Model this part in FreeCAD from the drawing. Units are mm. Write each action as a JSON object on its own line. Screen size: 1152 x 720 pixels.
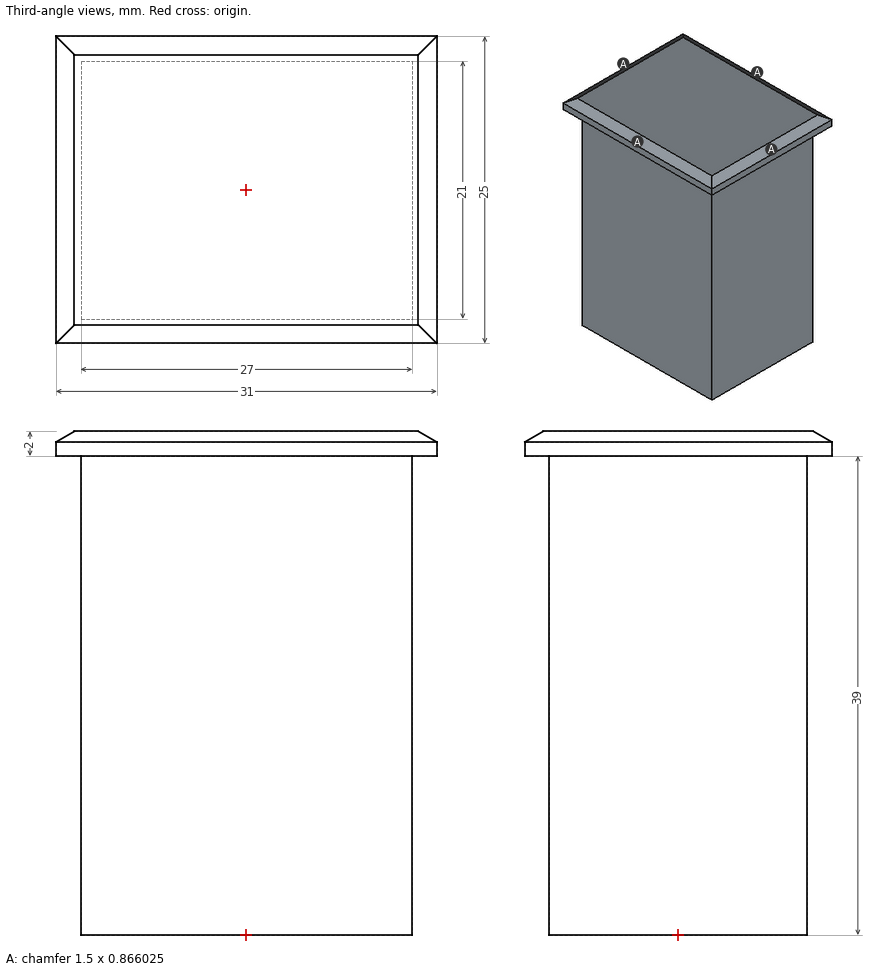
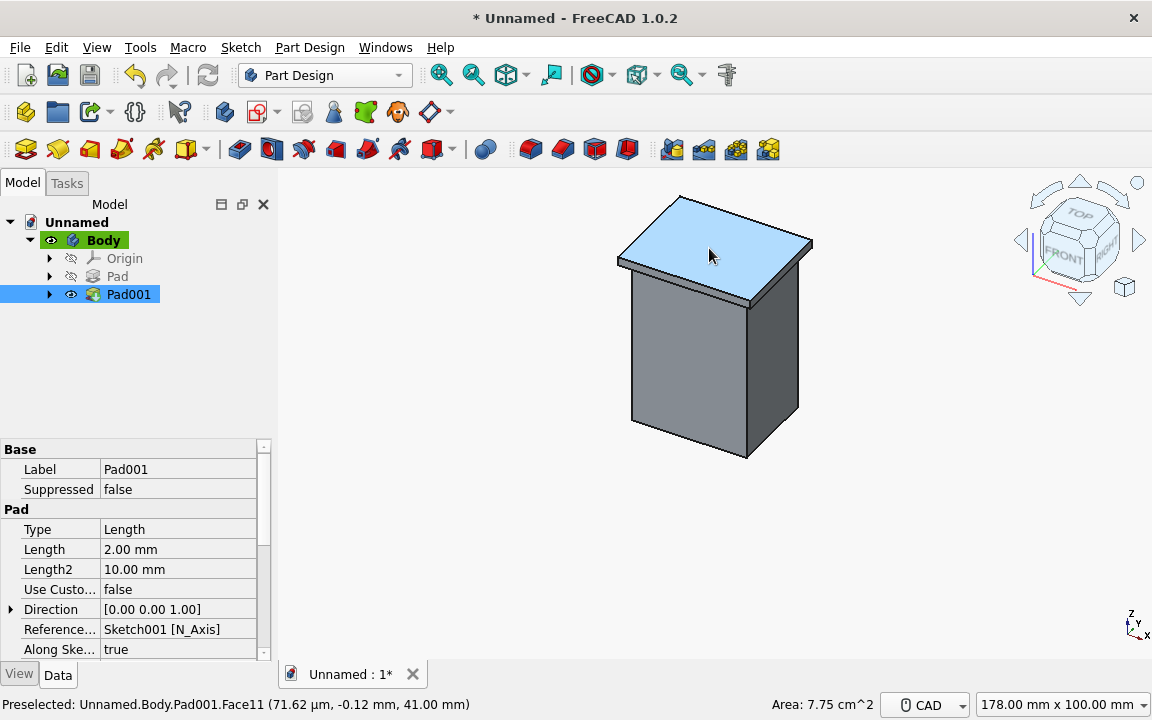
{"action": "left_click", "coordinate": [564, 150]}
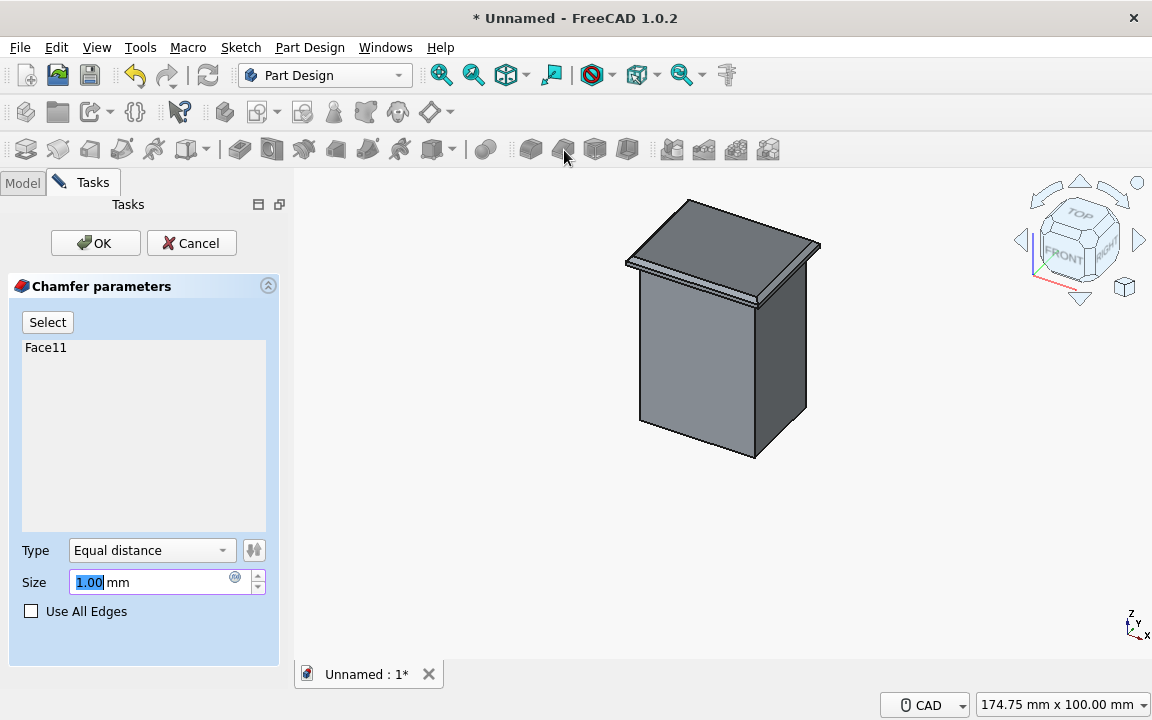
{"action": "type", "text": "1.5"}
{"action": "key", "text": "Tab"}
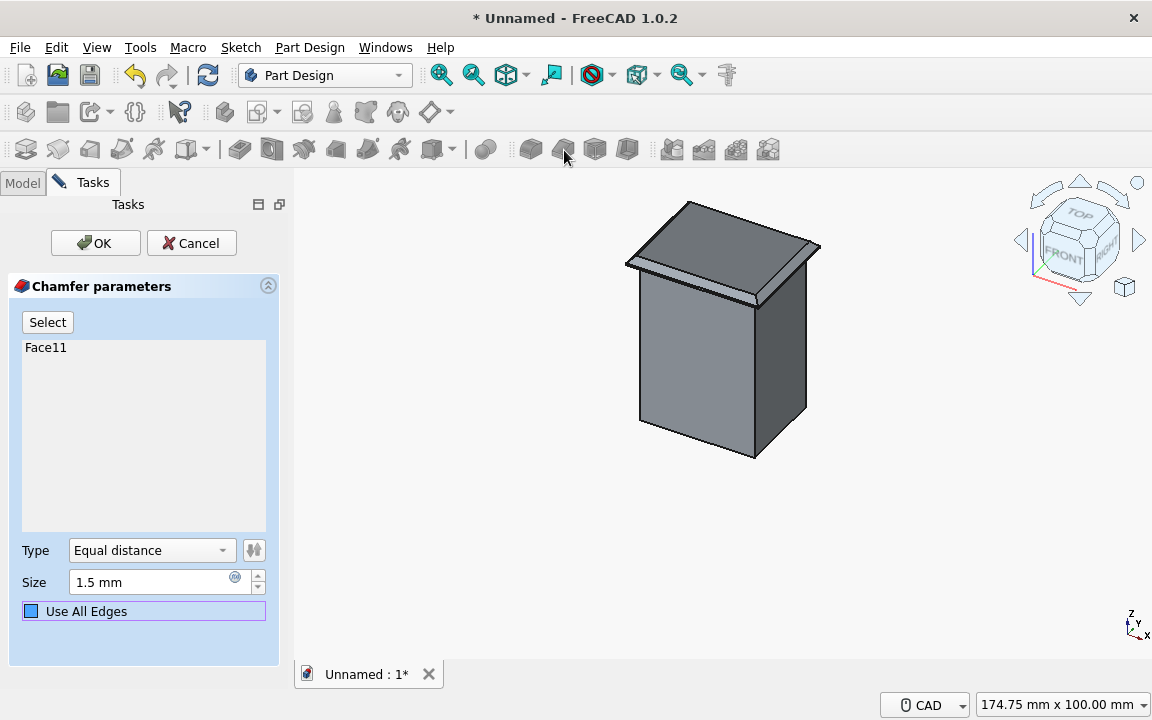
{"action": "left_click", "coordinate": [153, 550]}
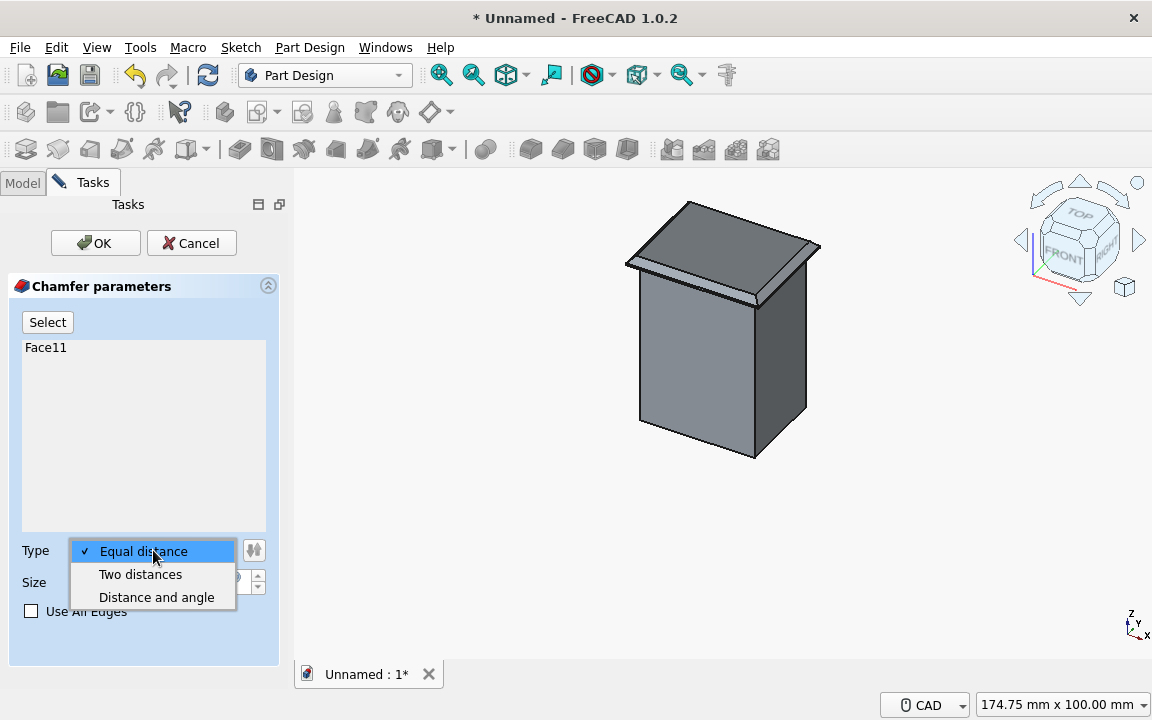
{"action": "left_click", "coordinate": [152, 574]}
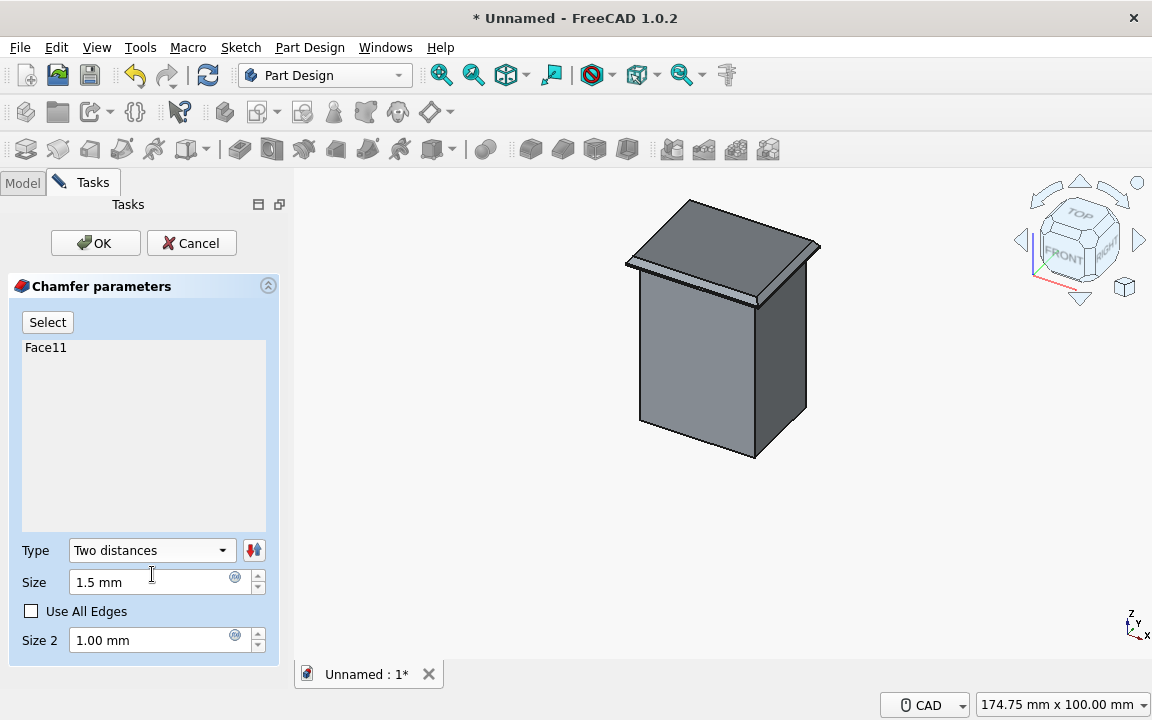
{"action": "triple_click", "coordinate": [160, 640]}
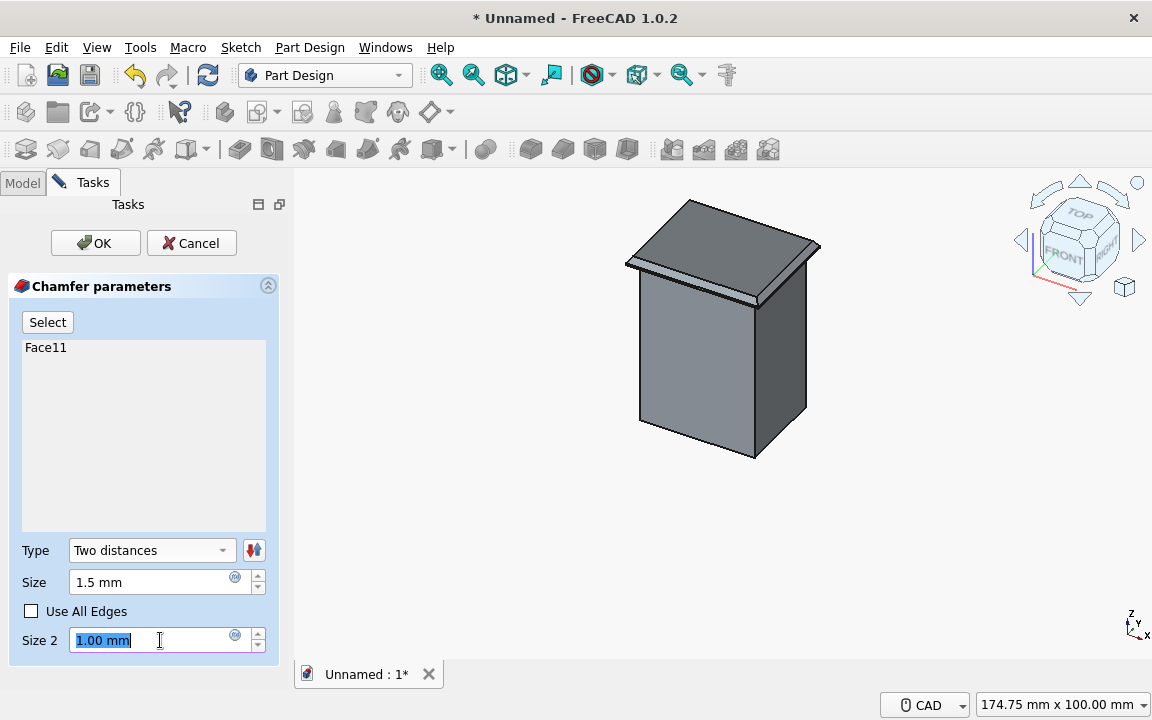
{"action": "type", "text": "0.866025"}
{"action": "key", "text": "Tab"}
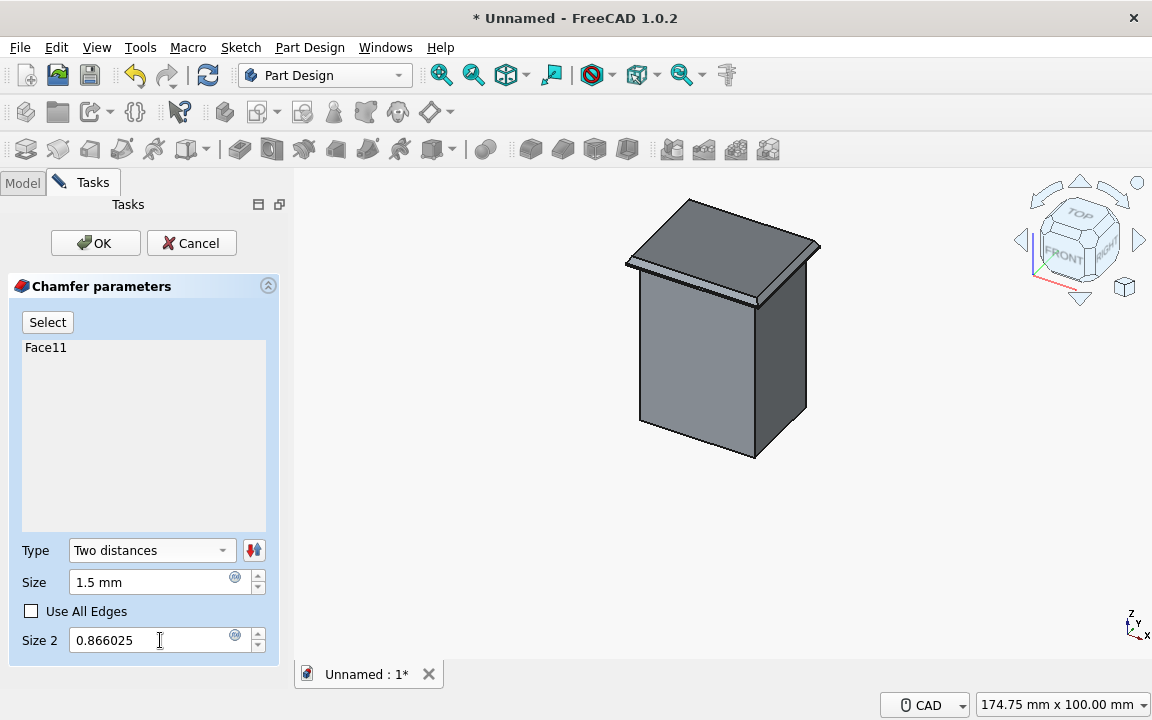
{"action": "left_click", "coordinate": [254, 550]}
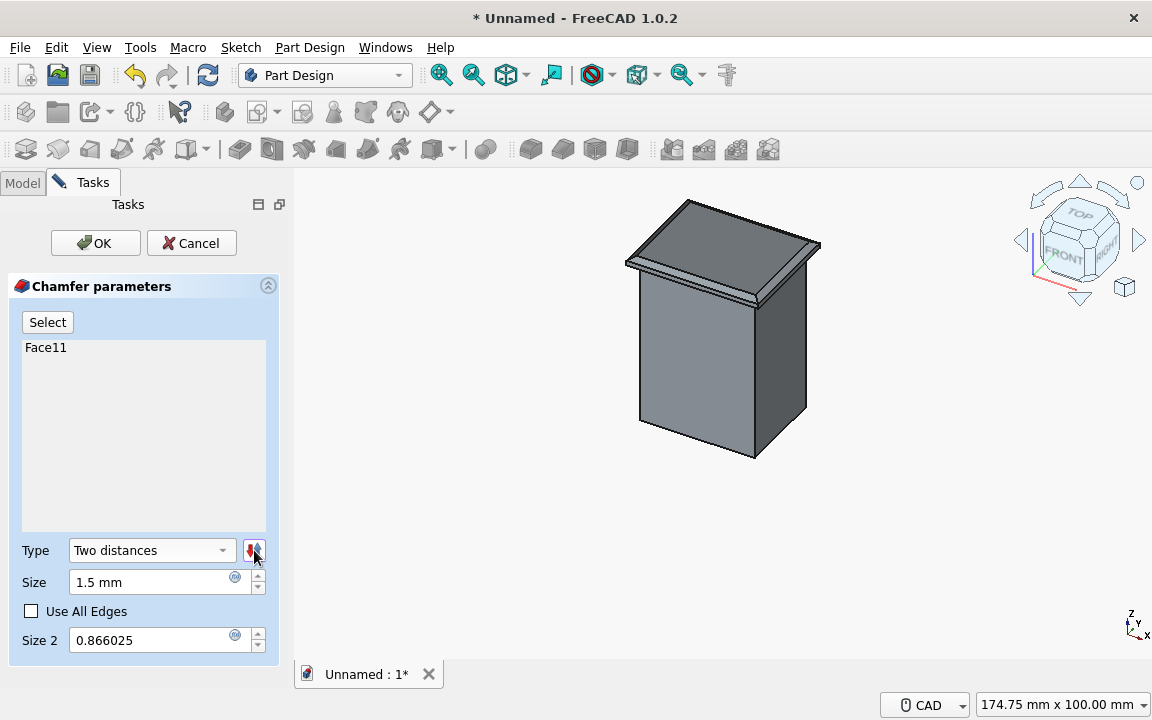
{"action": "left_click", "coordinate": [96, 243]}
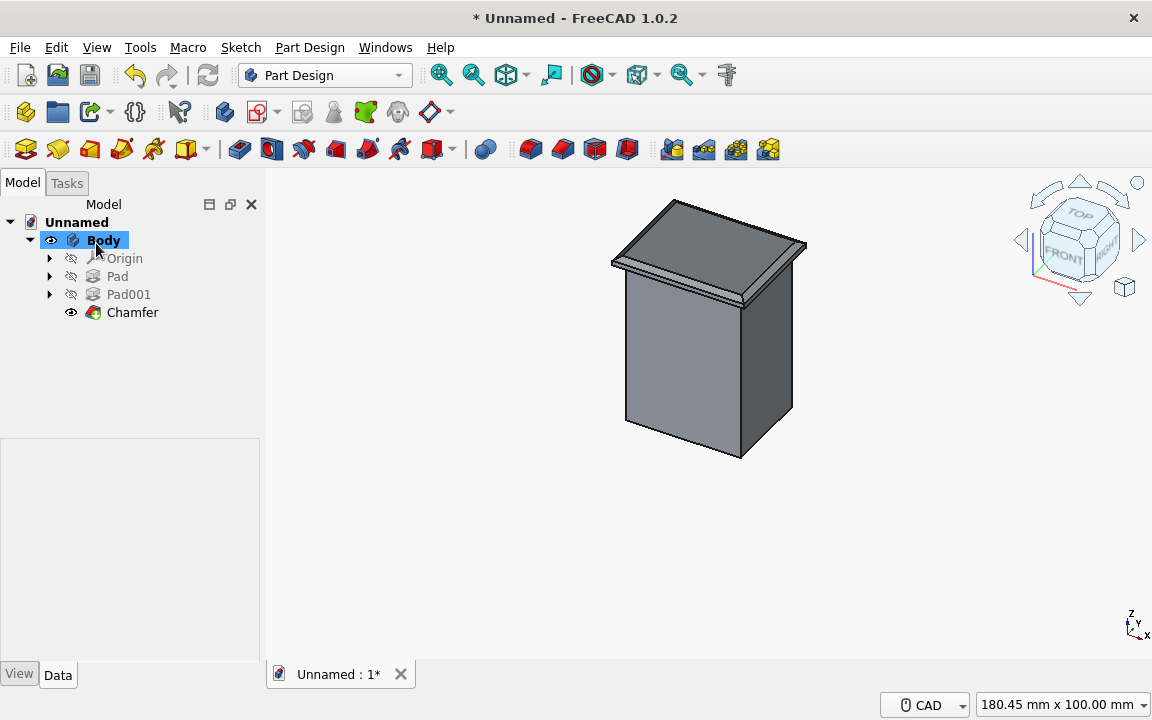
{"action": "key", "text": "0"}